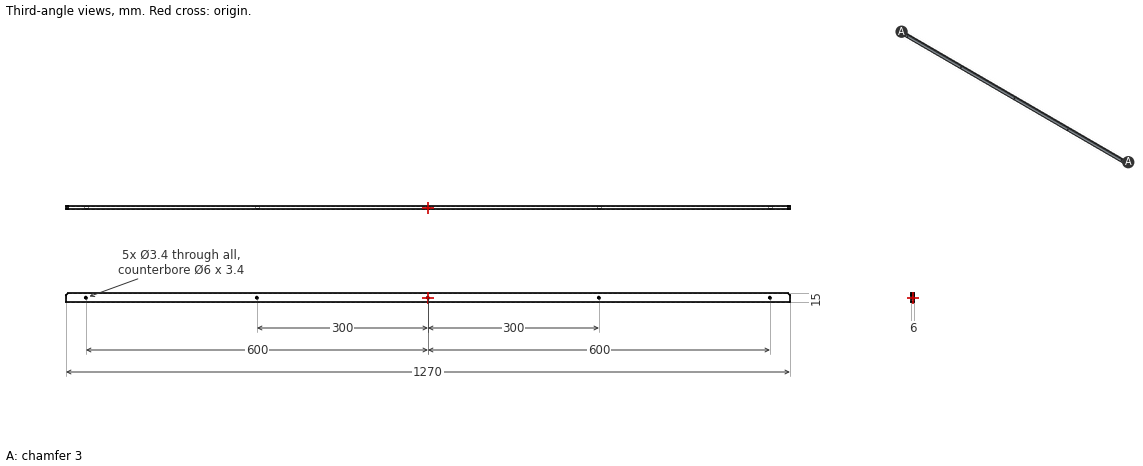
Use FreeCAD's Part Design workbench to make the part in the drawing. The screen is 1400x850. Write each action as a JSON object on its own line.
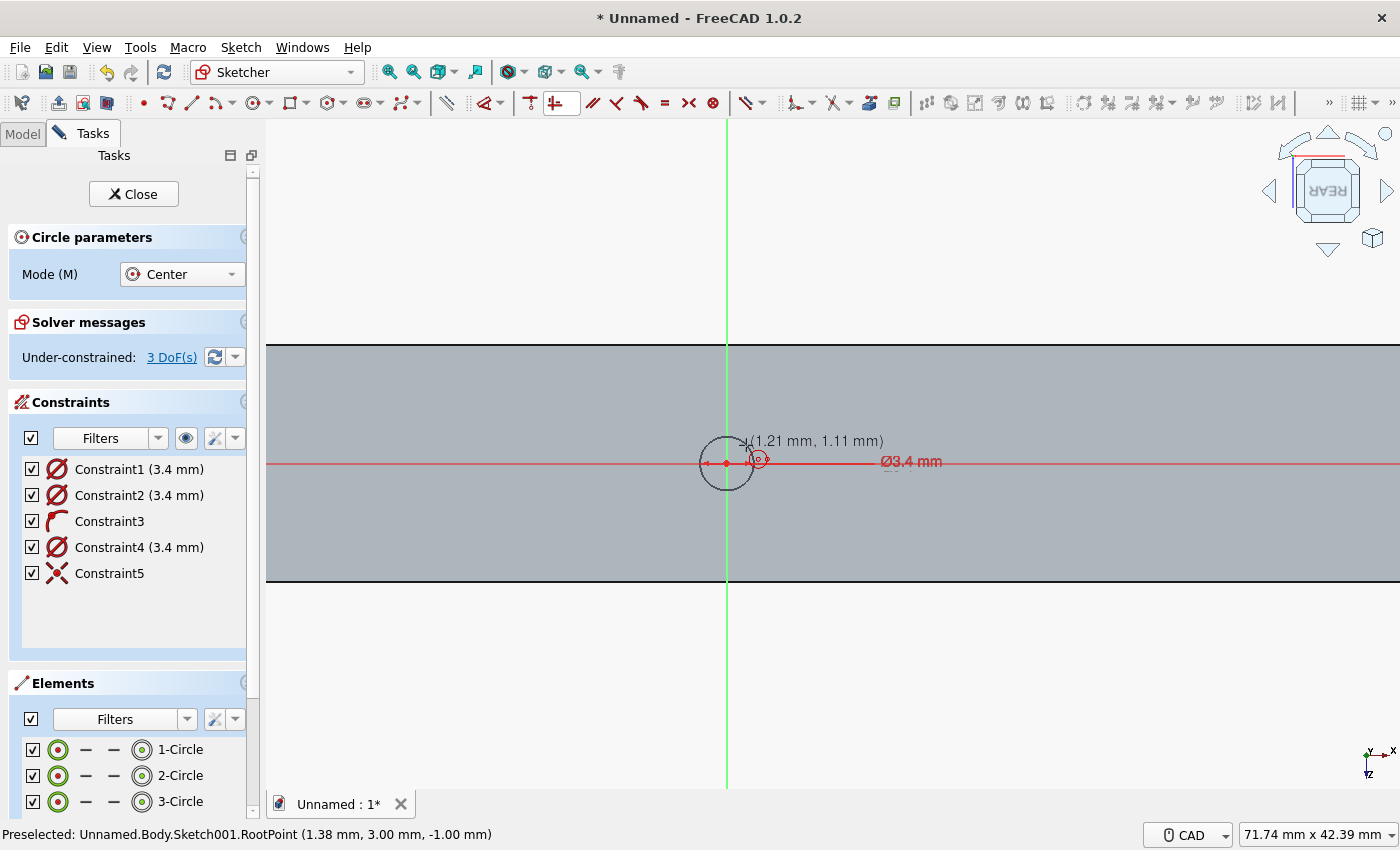
{"action": "scroll", "coordinate": [766, 454], "scroll_direction": "down", "scroll_amount": 16}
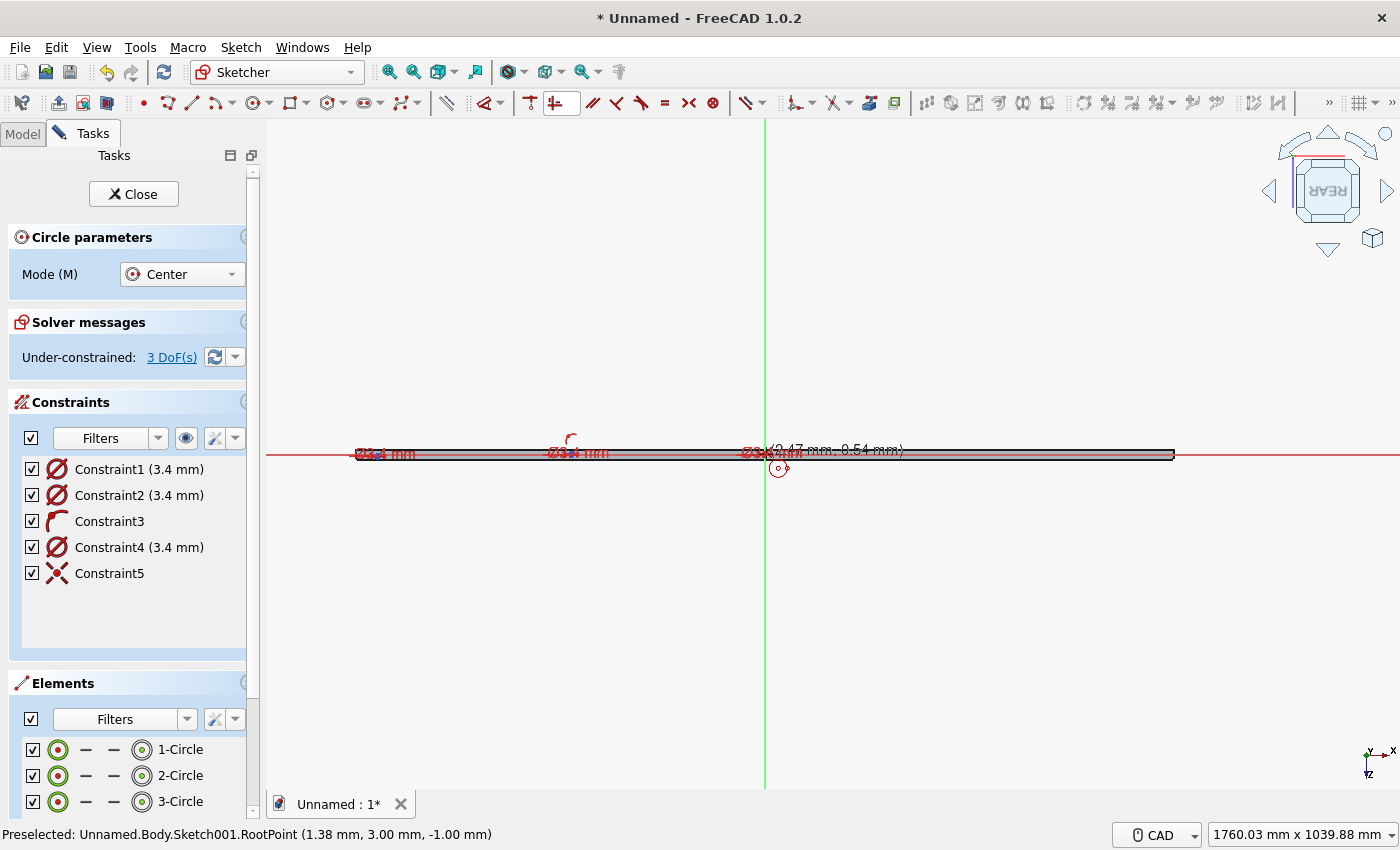
{"action": "scroll", "coordinate": [958, 455], "scroll_direction": "up", "scroll_amount": 16}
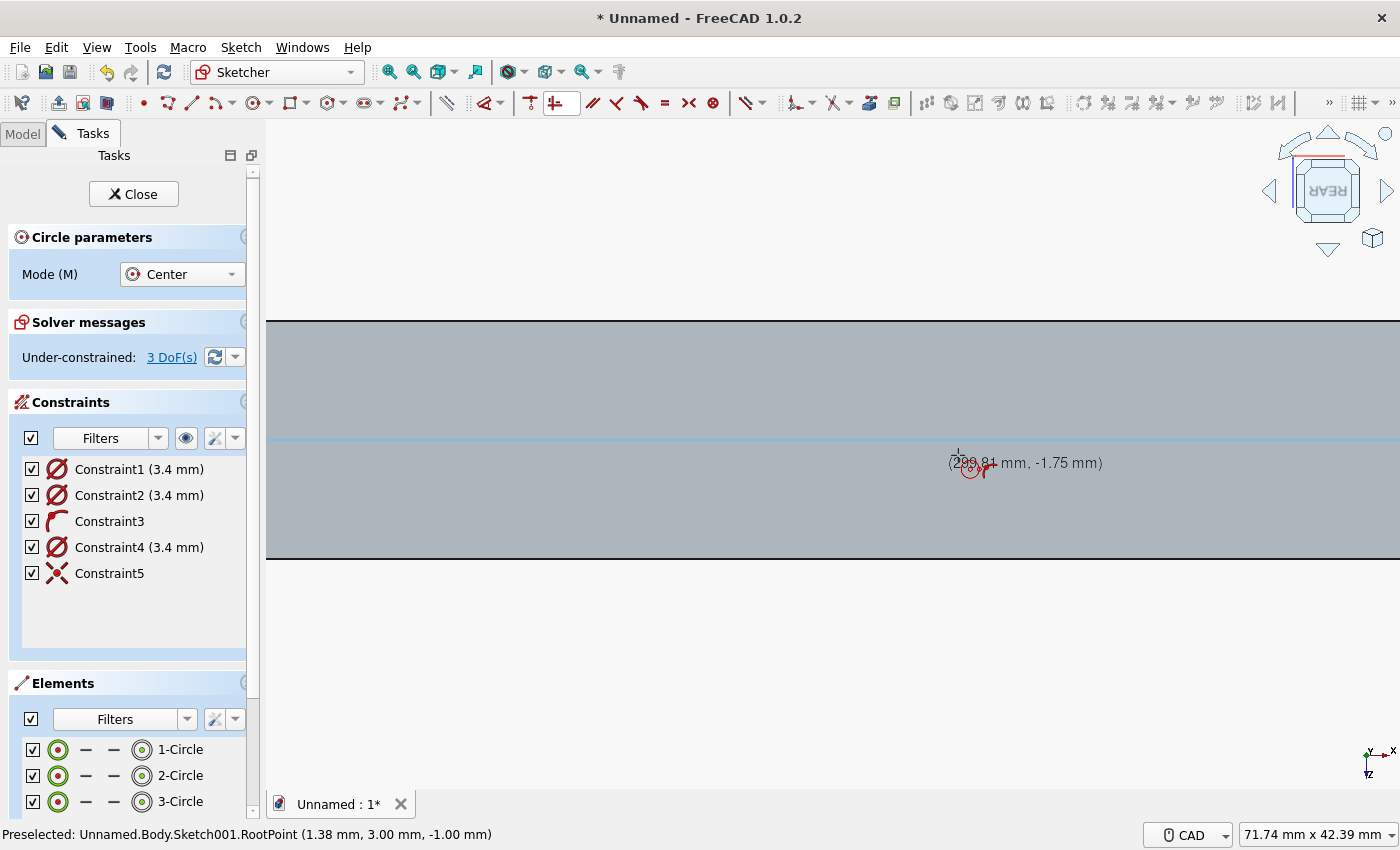
{"action": "scroll", "coordinate": [958, 455], "scroll_direction": "down", "scroll_amount": 16}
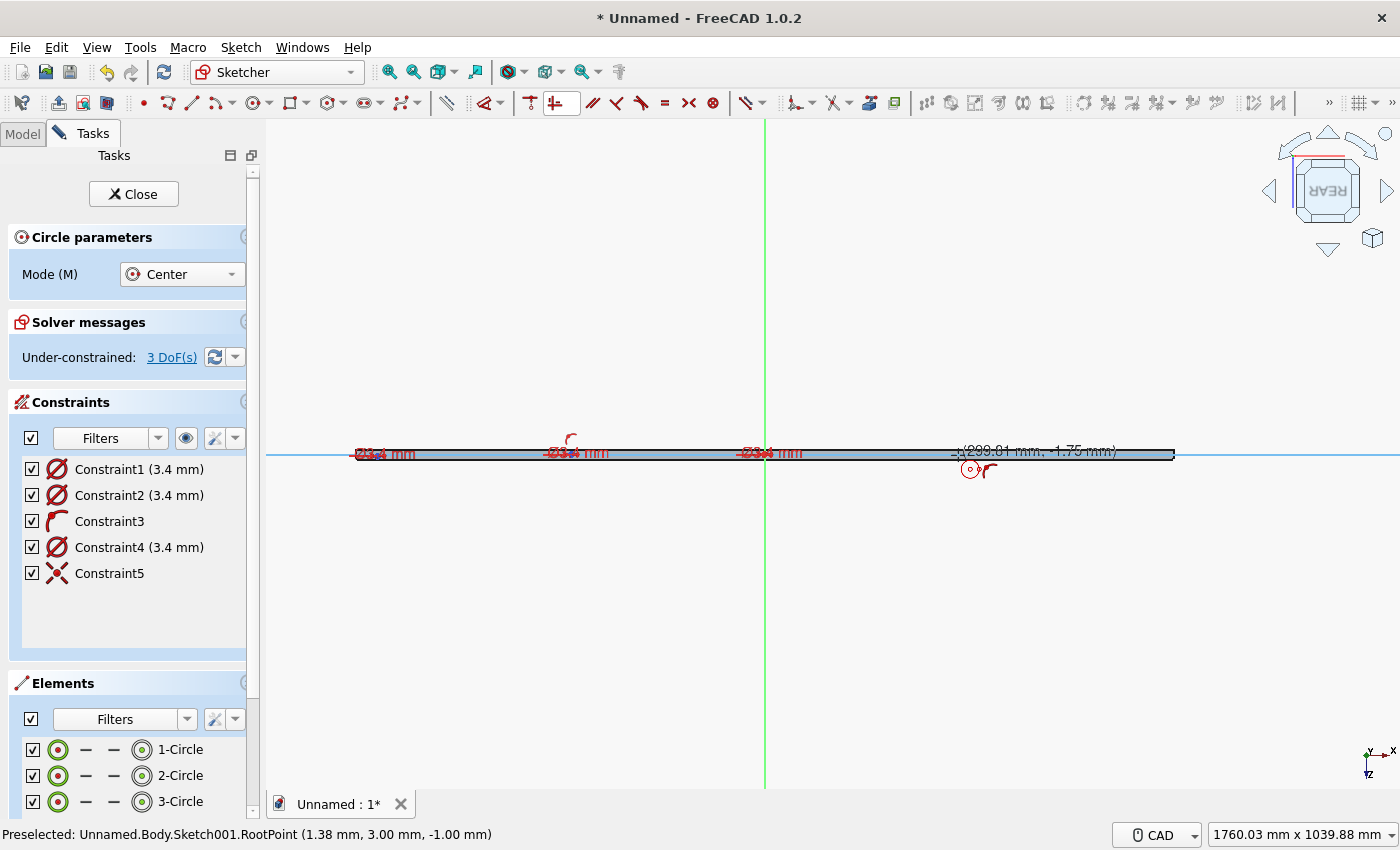
{"action": "left_click", "coordinate": [958, 455]}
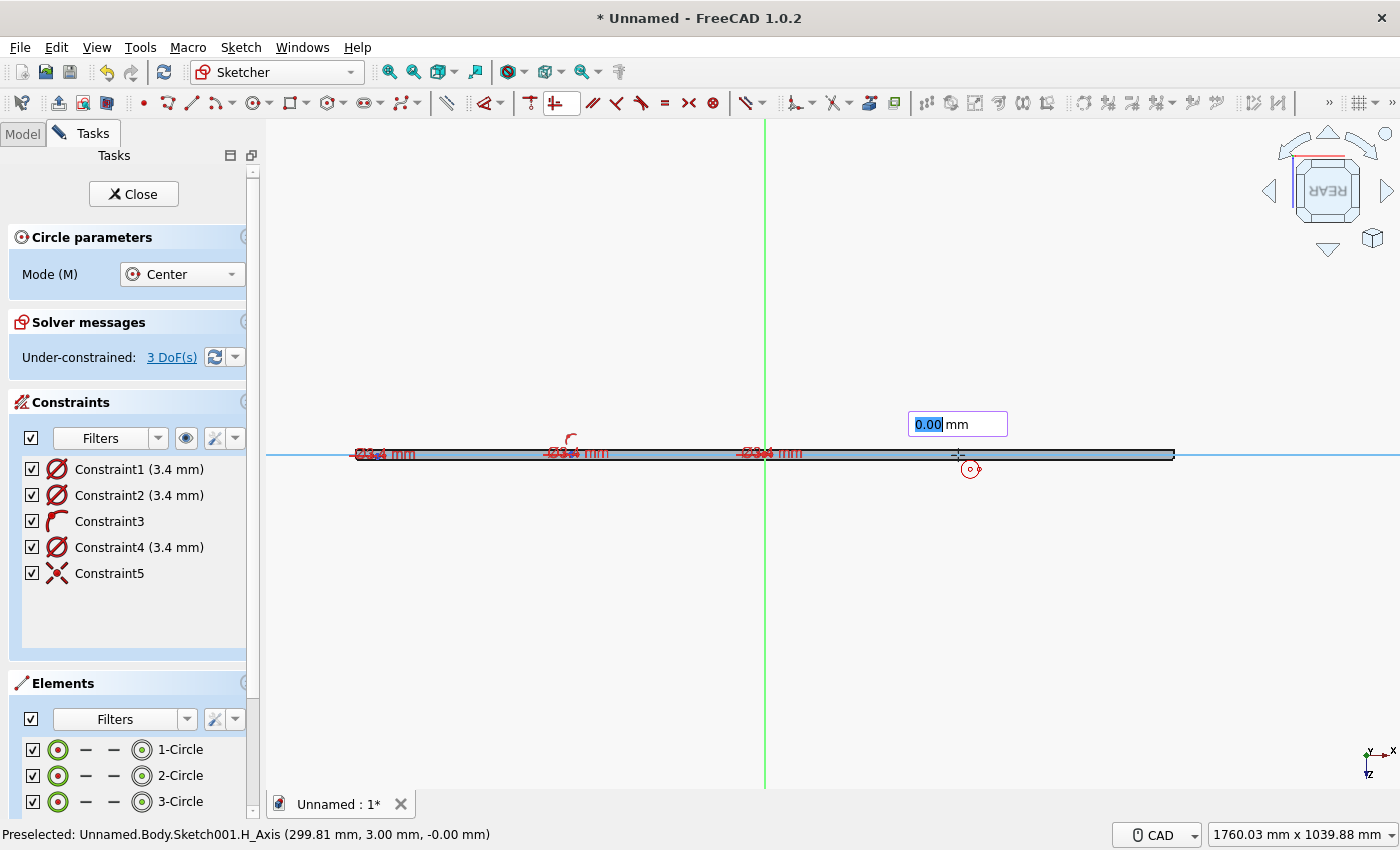
{"action": "scroll", "coordinate": [958, 456], "scroll_direction": "up", "scroll_amount": 14}
{"action": "mouse_move", "coordinate": [944, 447]}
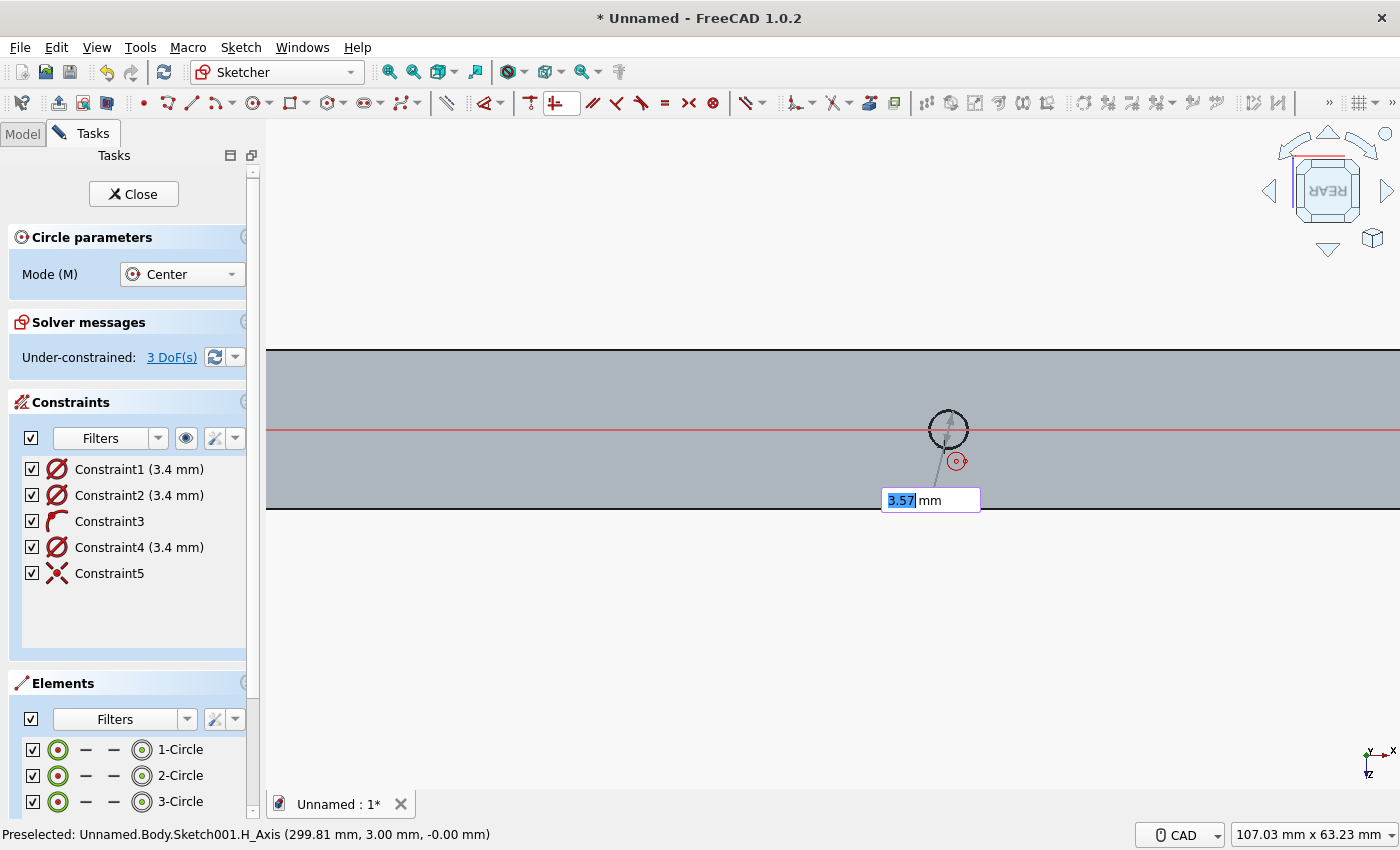
{"action": "type", "text": "3.4"}
{"action": "key", "text": "Return"}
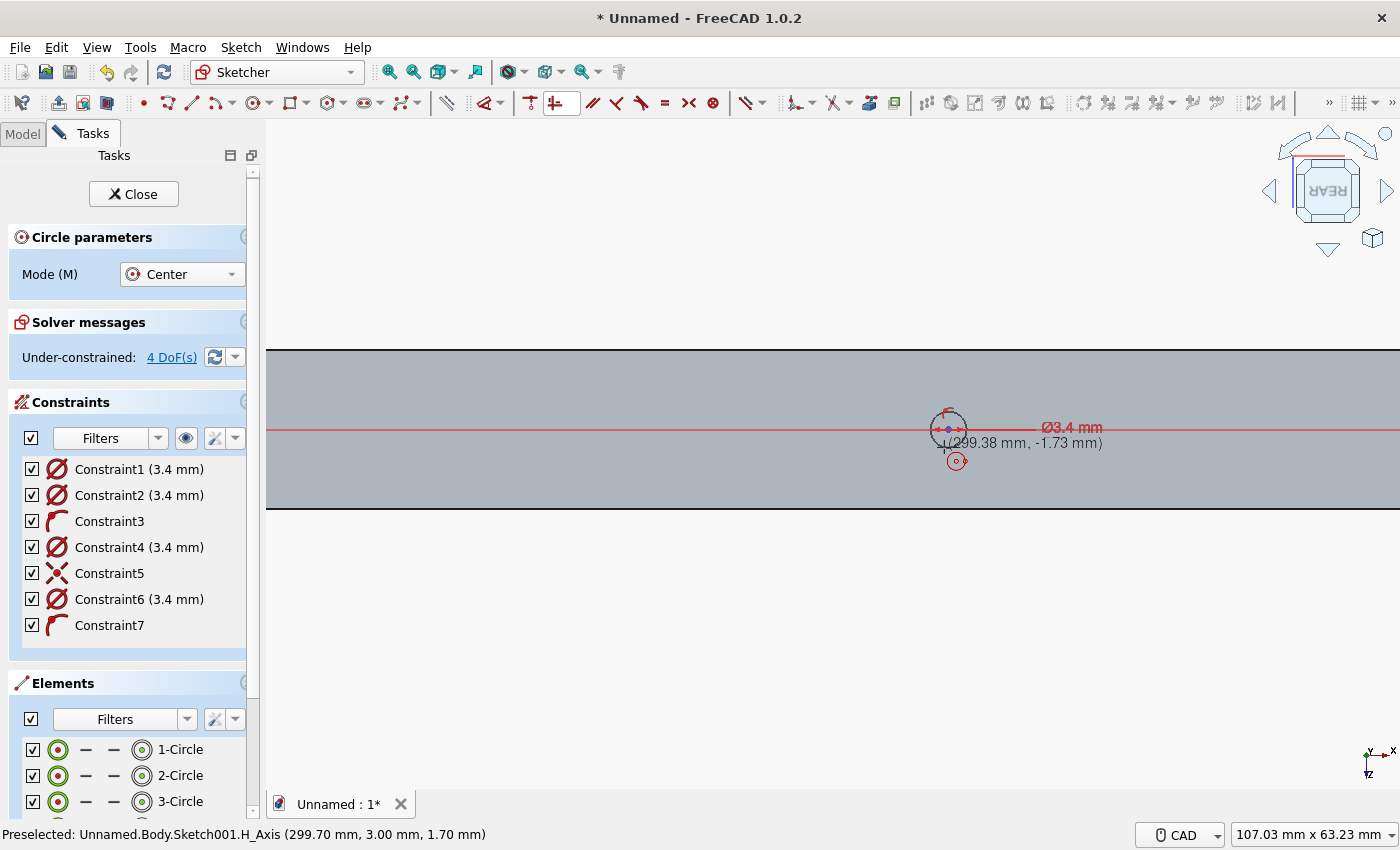
{"action": "scroll", "coordinate": [921, 455], "scroll_direction": "down", "scroll_amount": 15}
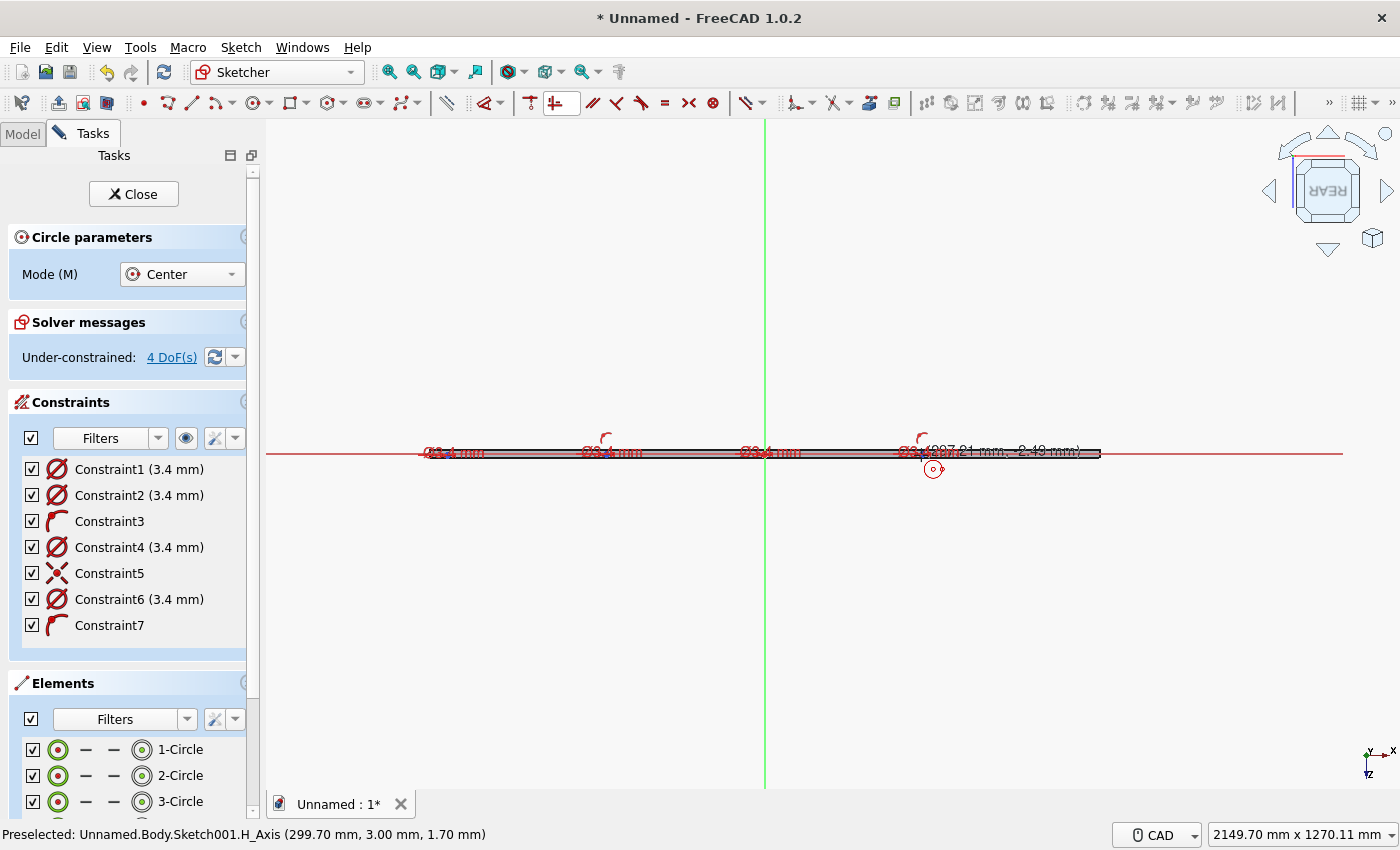
{"action": "scroll", "coordinate": [1081, 454], "scroll_direction": "up", "scroll_amount": 17}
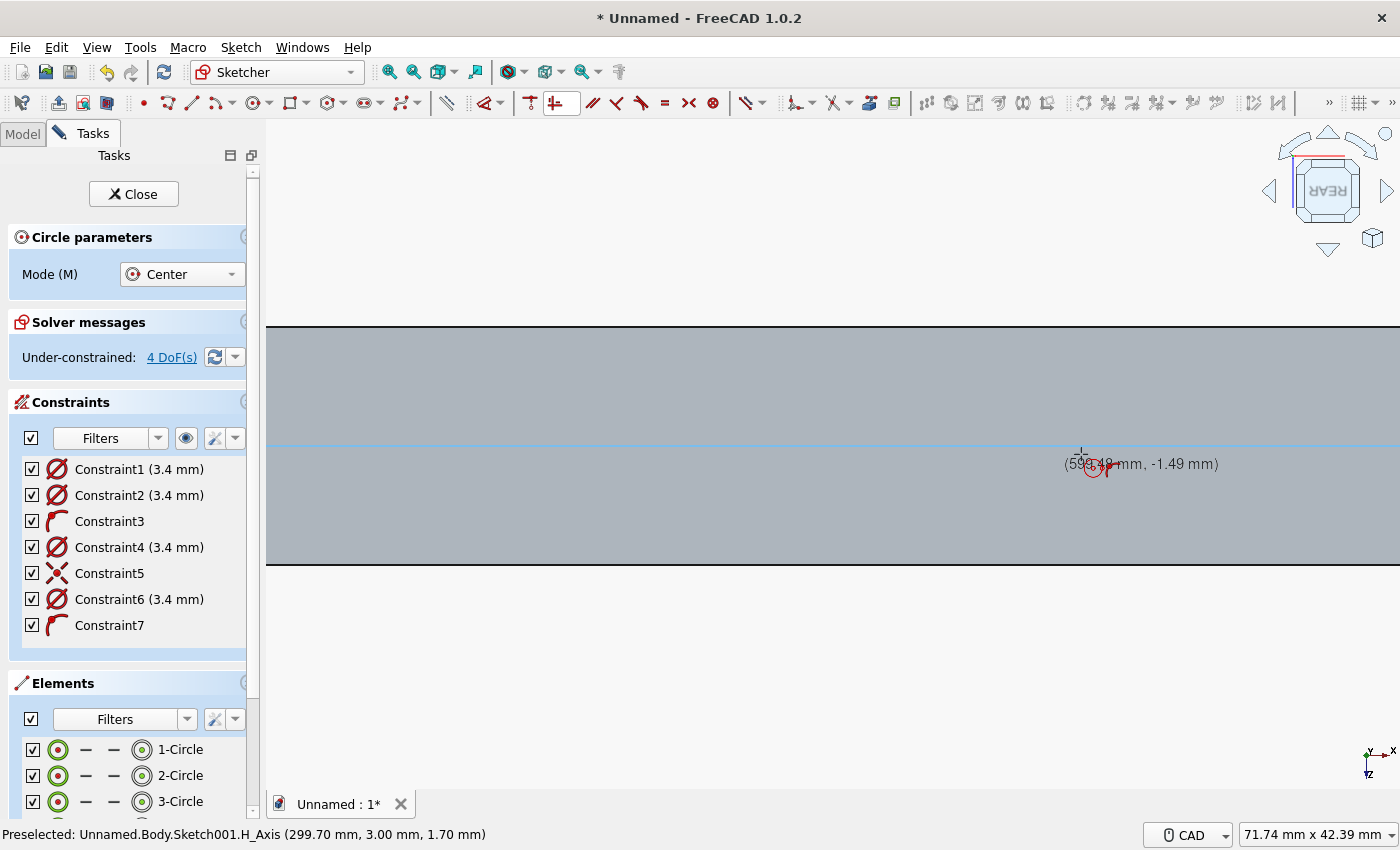
{"action": "scroll", "coordinate": [1155, 454], "scroll_direction": "down", "scroll_amount": 16}